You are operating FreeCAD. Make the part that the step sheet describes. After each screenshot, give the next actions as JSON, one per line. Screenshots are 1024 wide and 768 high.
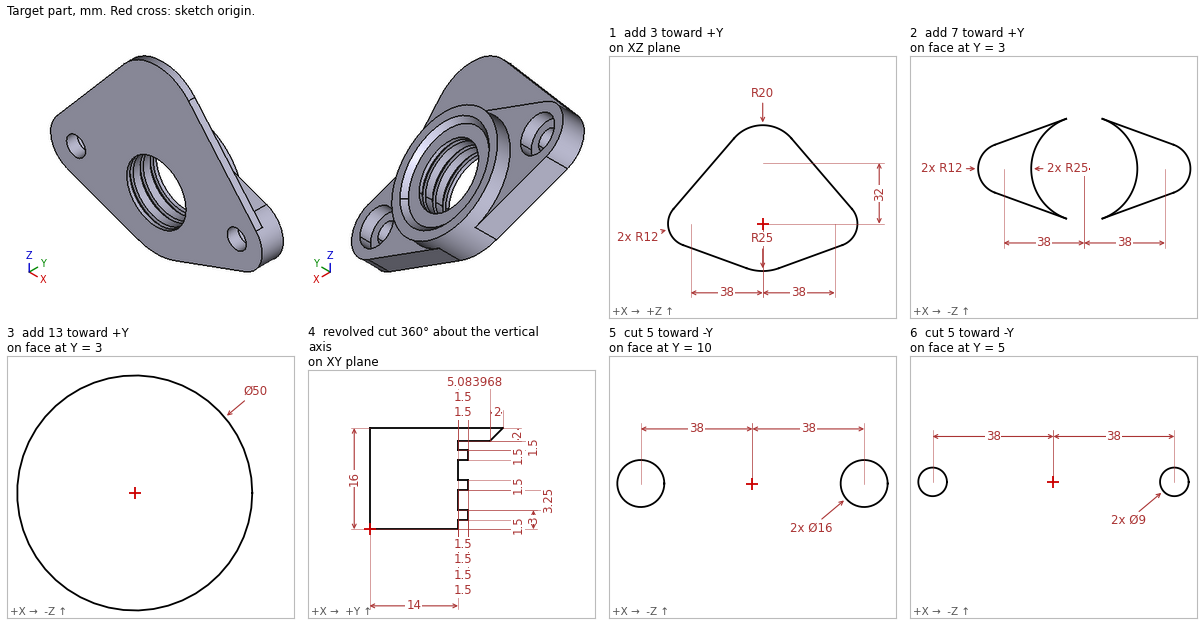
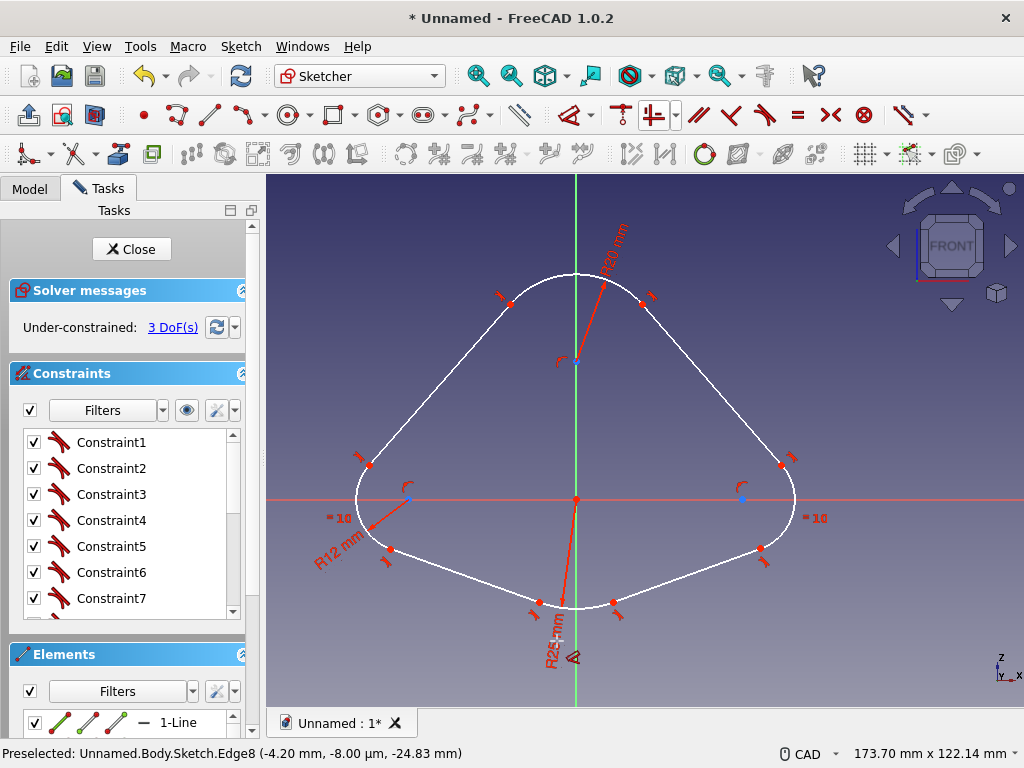
{"action": "left_click", "coordinate": [409, 500]}
{"action": "left_click", "coordinate": [492, 534]}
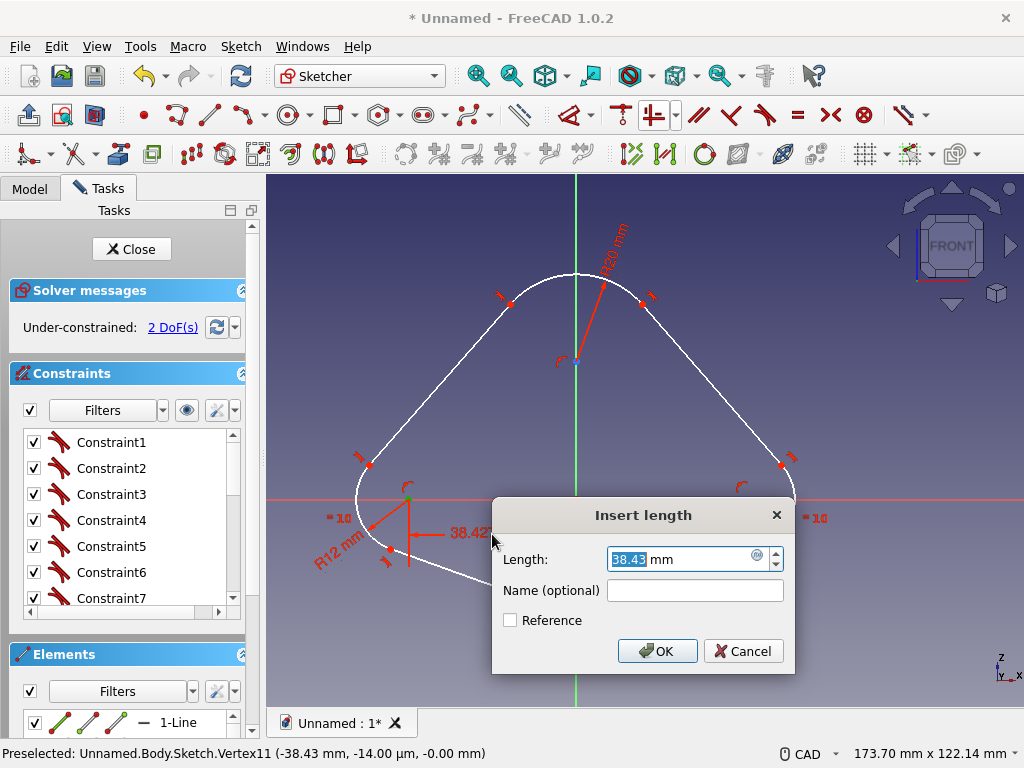
{"action": "type", "text": "38"}
{"action": "key", "text": "Return"}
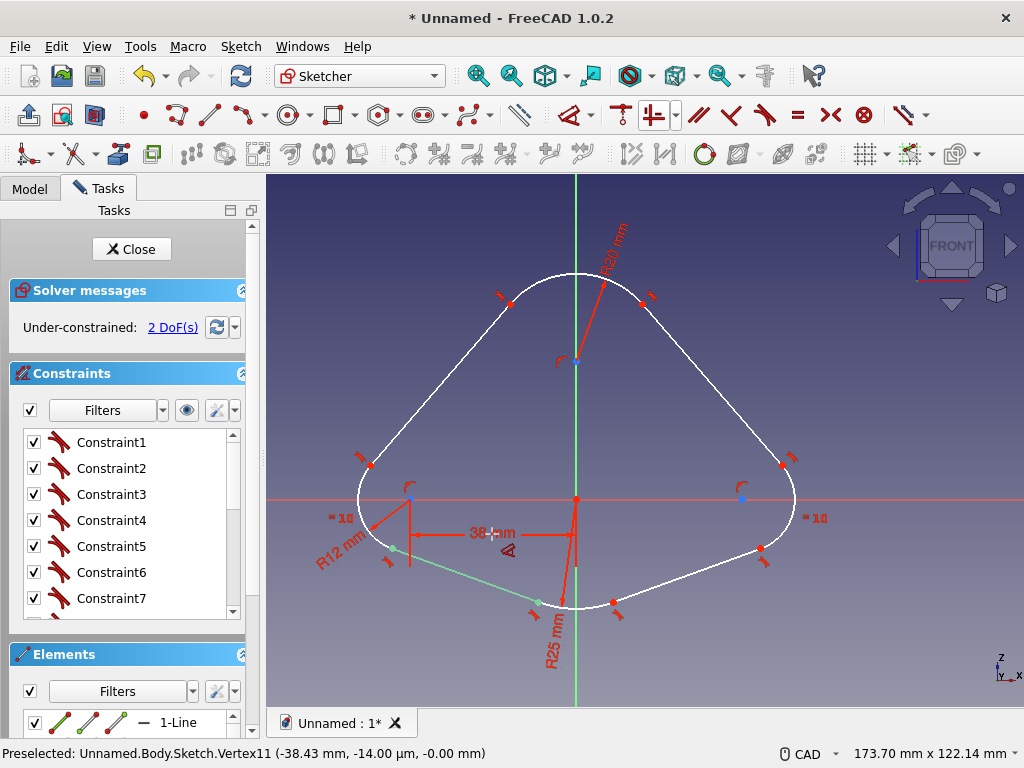
{"action": "left_click", "coordinate": [576, 361]}
{"action": "left_click", "coordinate": [610, 430]}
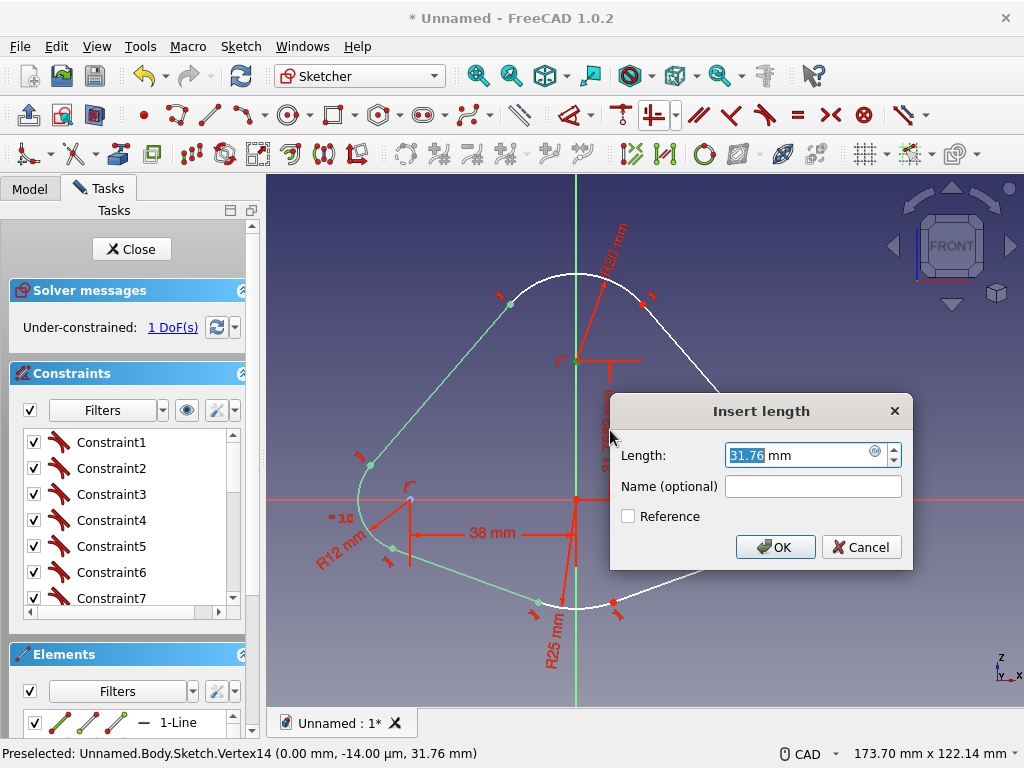
{"action": "type", "text": "32"}
{"action": "key", "text": "Return"}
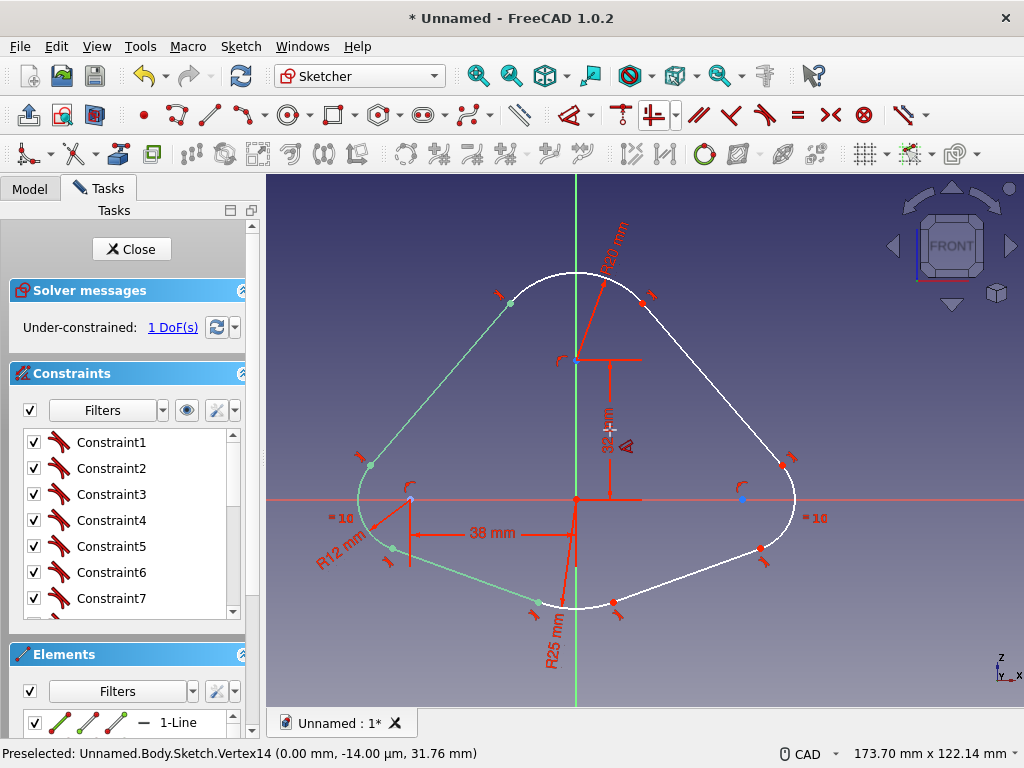
{"action": "left_click", "coordinate": [742, 500]}
{"action": "left_click", "coordinate": [659, 534]}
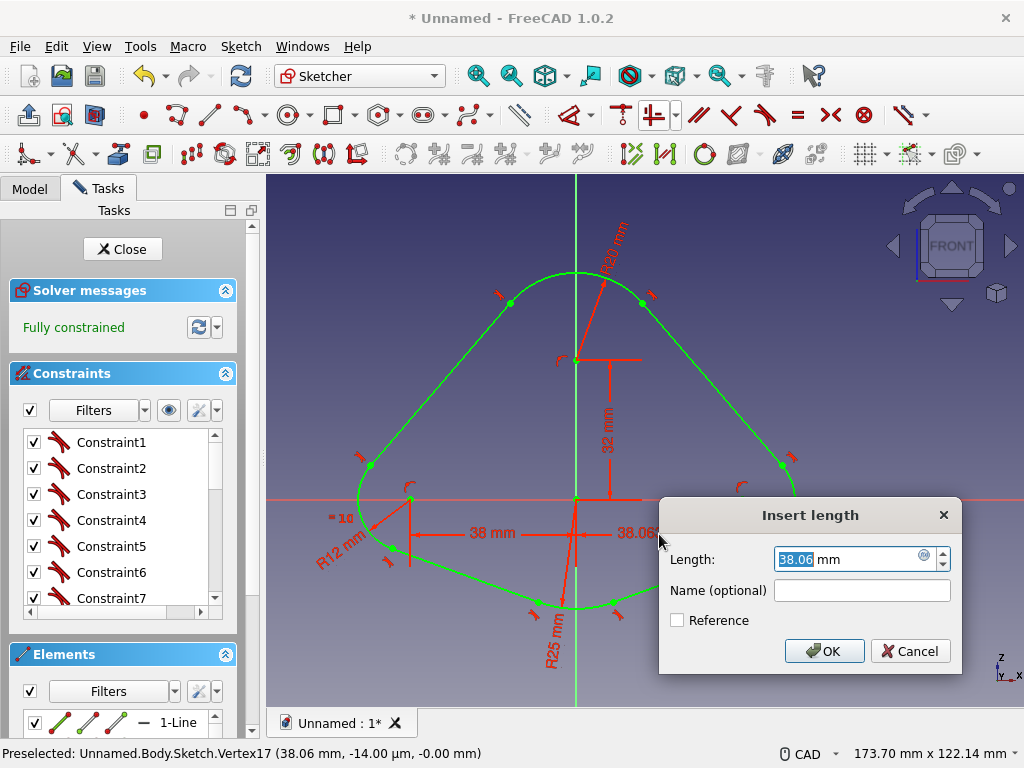
{"action": "type", "text": "38"}
{"action": "key", "text": "Return"}
{"action": "key", "text": "Escape"}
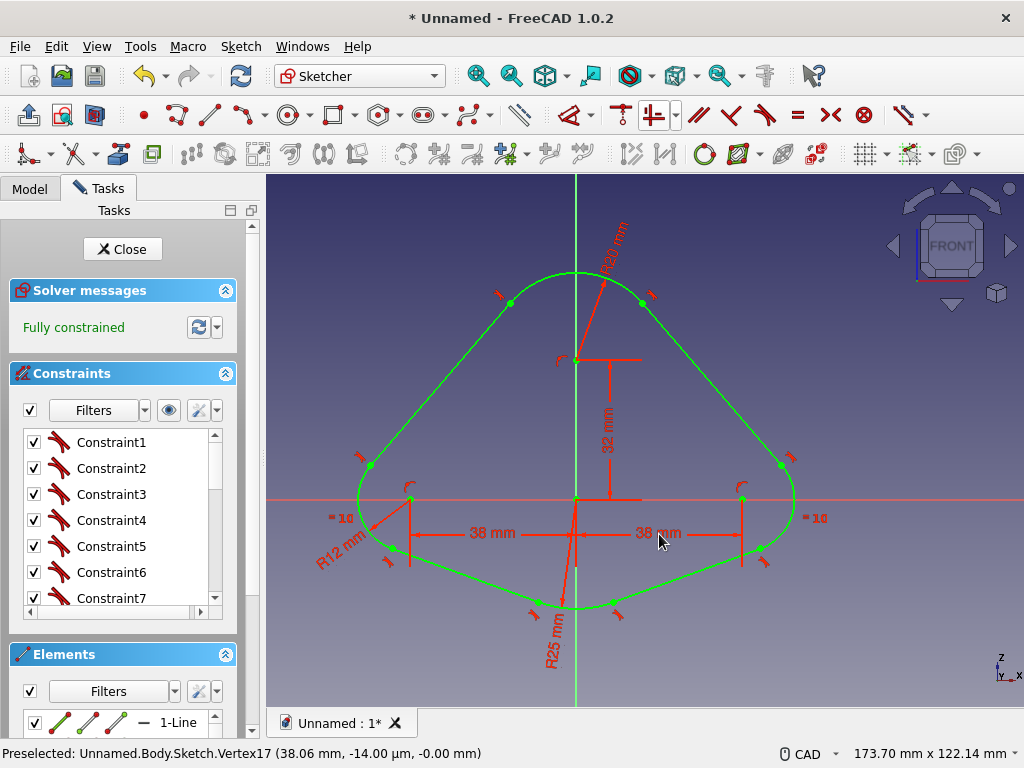
{"action": "left_click", "coordinate": [123, 249]}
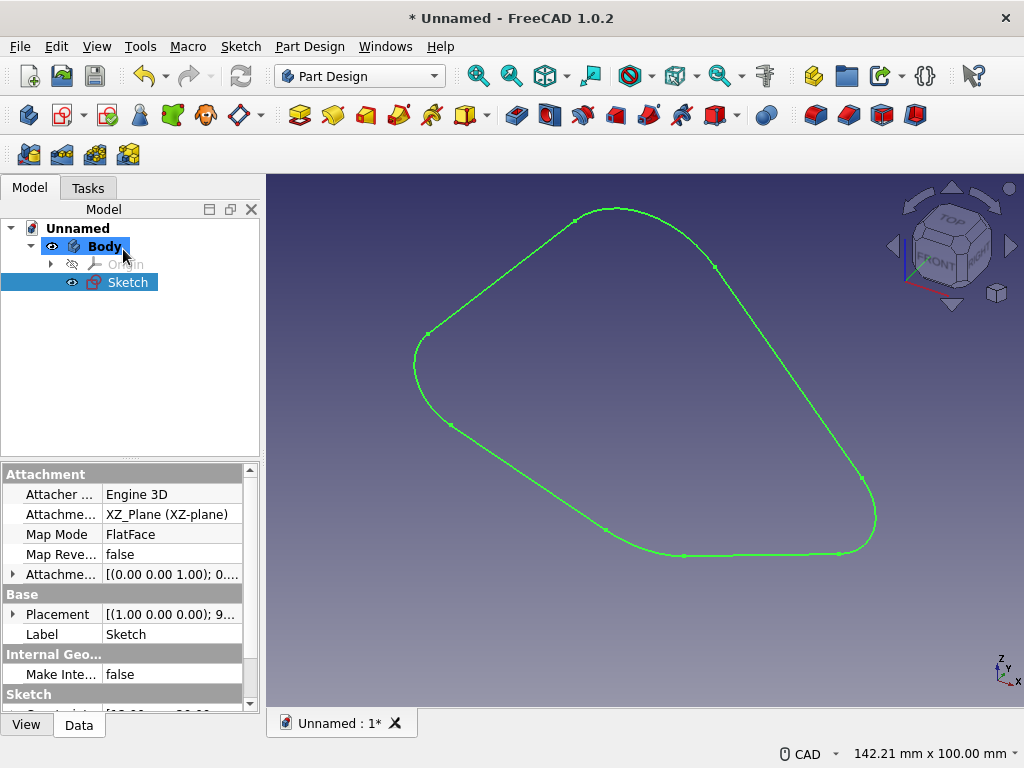
{"action": "left_click", "coordinate": [300, 116]}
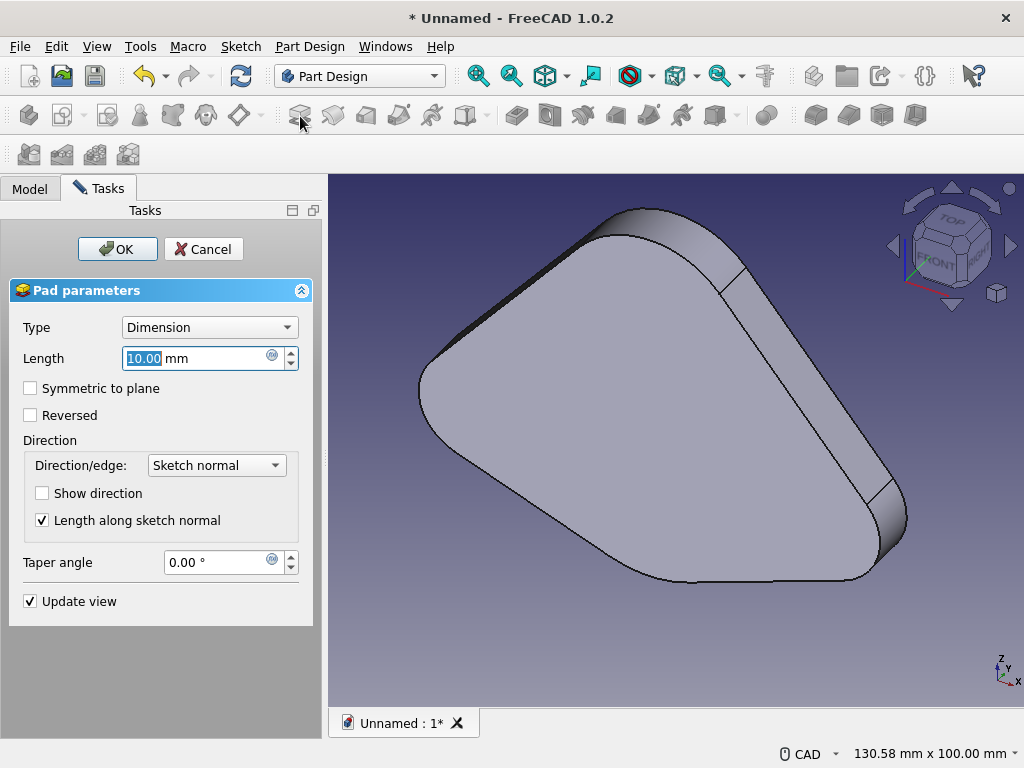
{"action": "type", "text": "3"}
{"action": "key", "text": "Tab"}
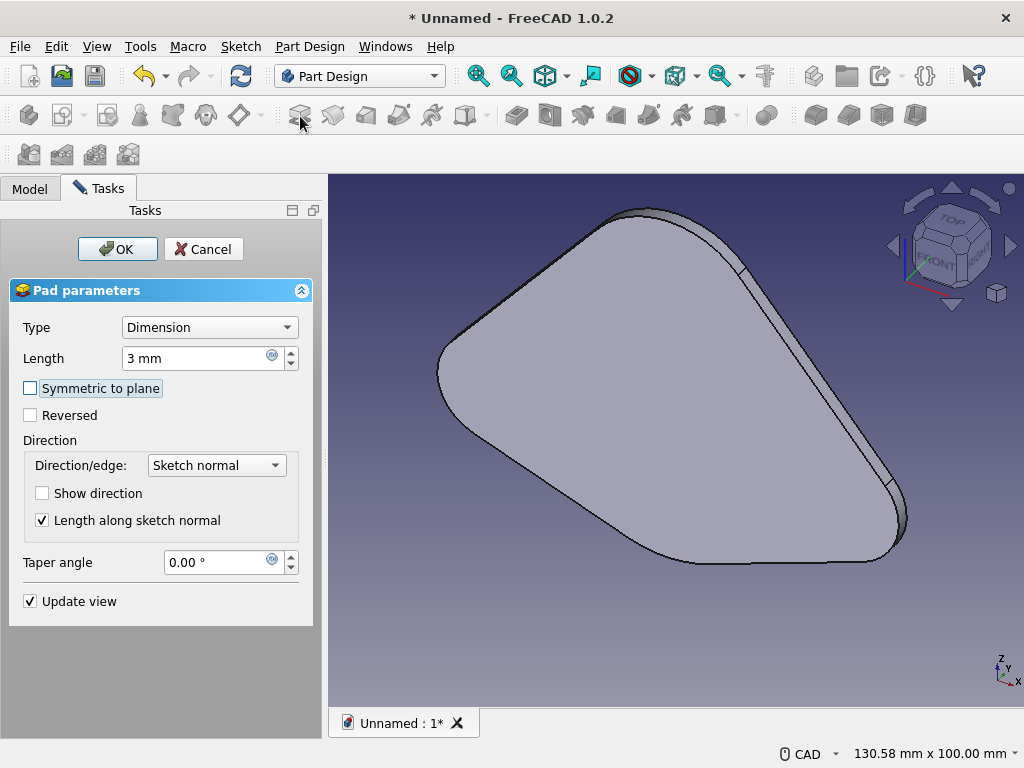
{"action": "left_click", "coordinate": [31, 415]}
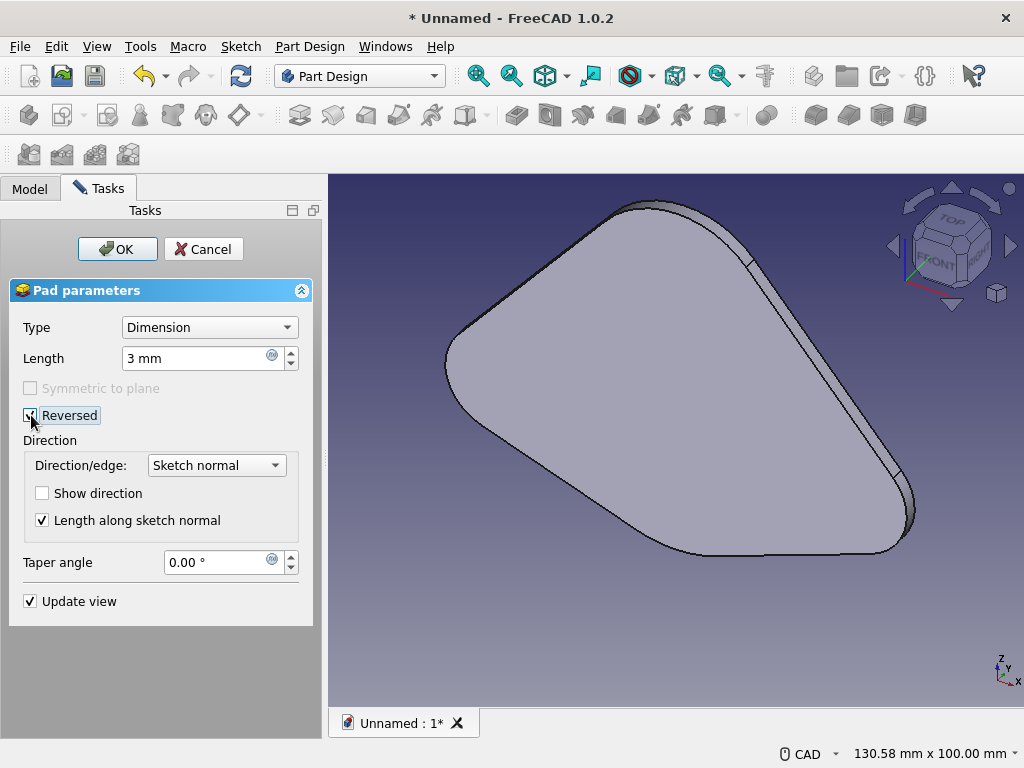
{"action": "left_click", "coordinate": [118, 249]}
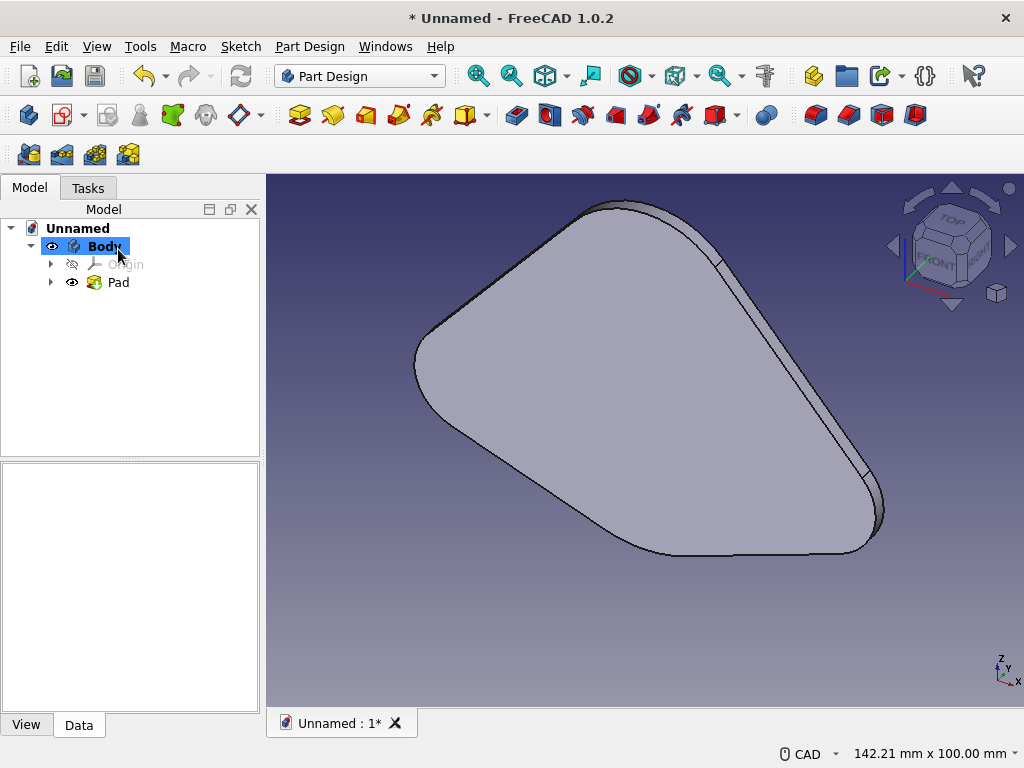
{"action": "left_click", "coordinate": [479, 76]}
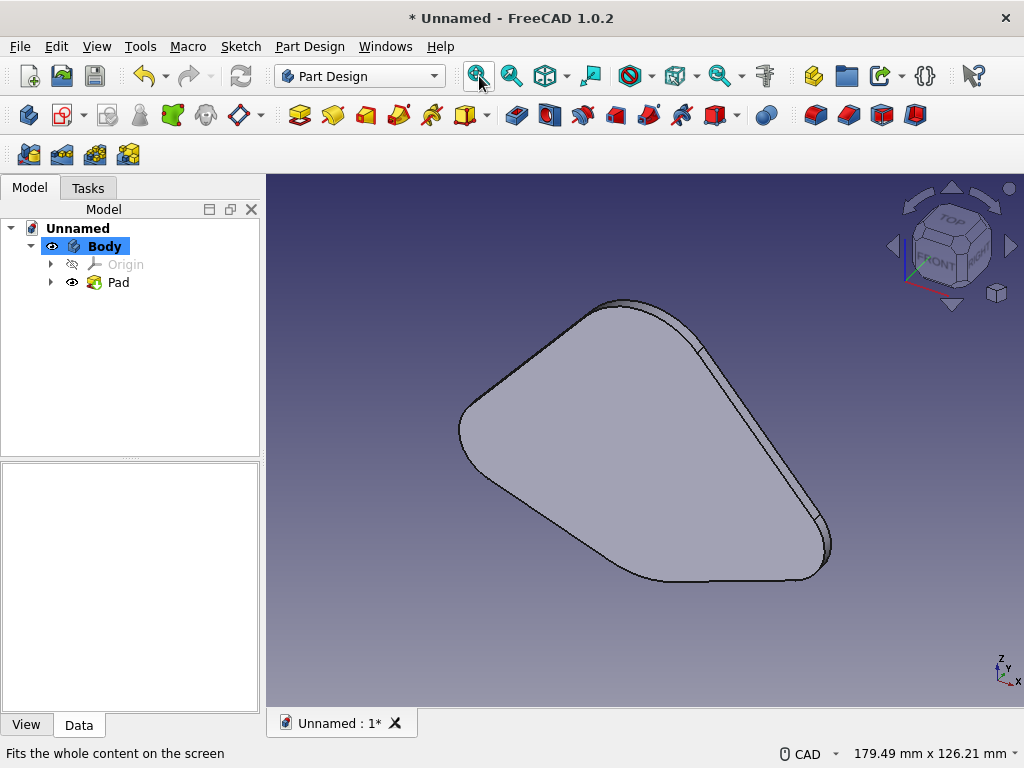
{"action": "key", "text": "4"}